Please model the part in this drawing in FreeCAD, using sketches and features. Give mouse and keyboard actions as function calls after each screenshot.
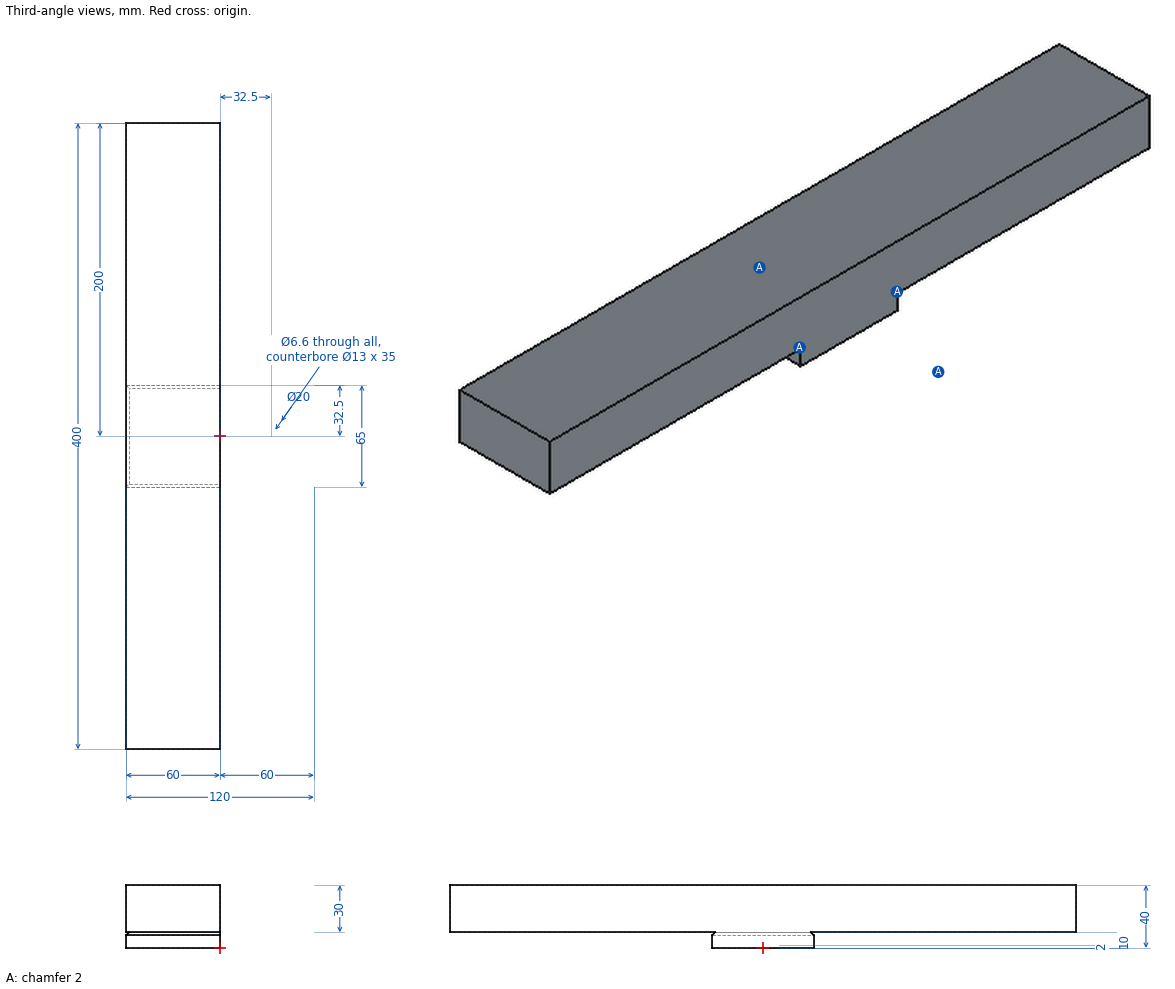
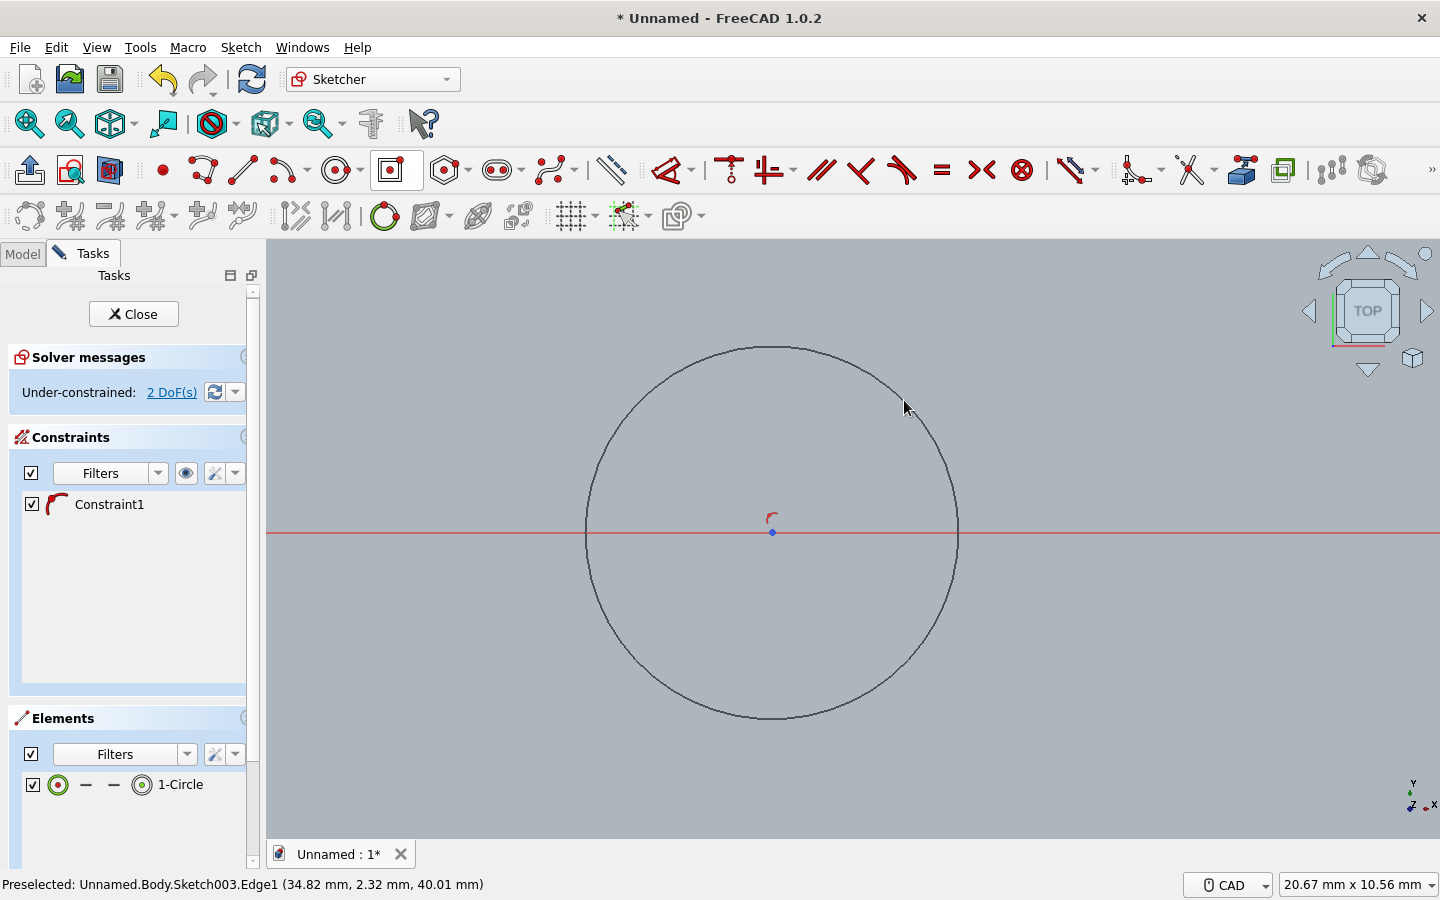
click(666, 170)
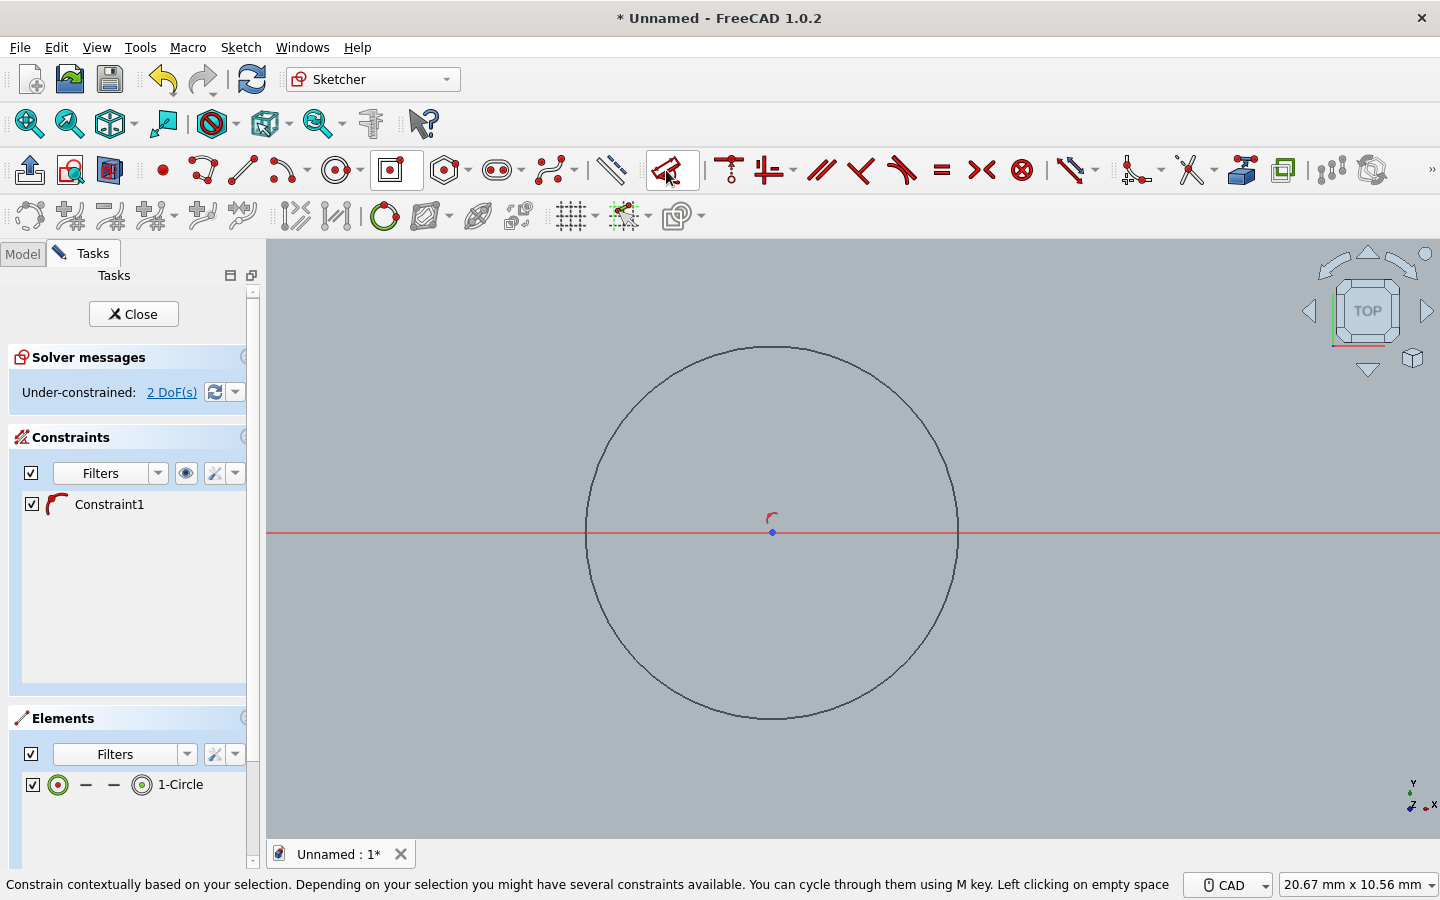
click(903, 400)
click(925, 377)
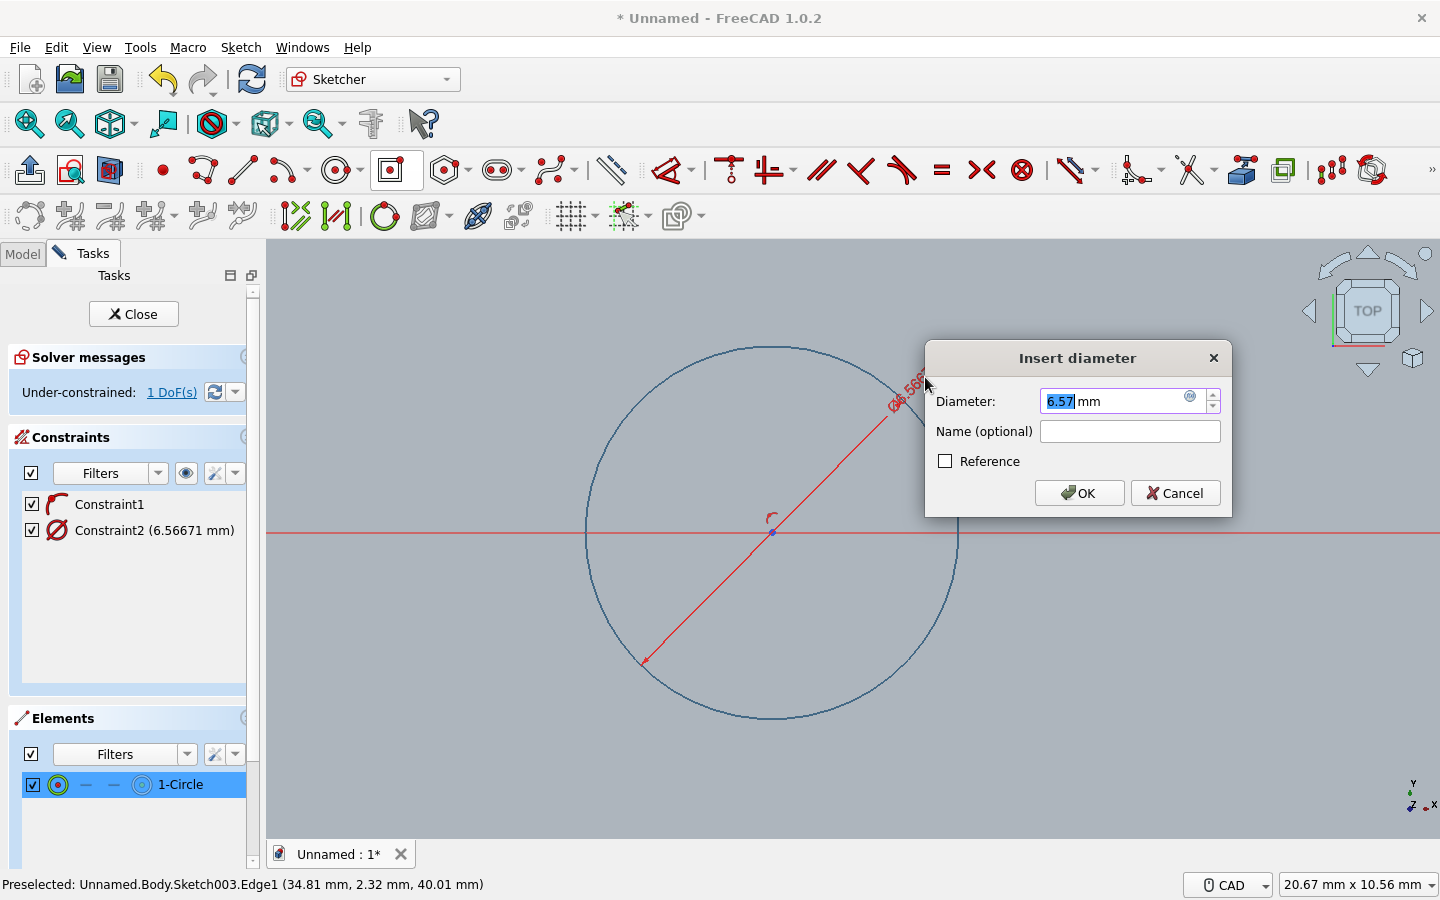
text(6.6)
key(Return)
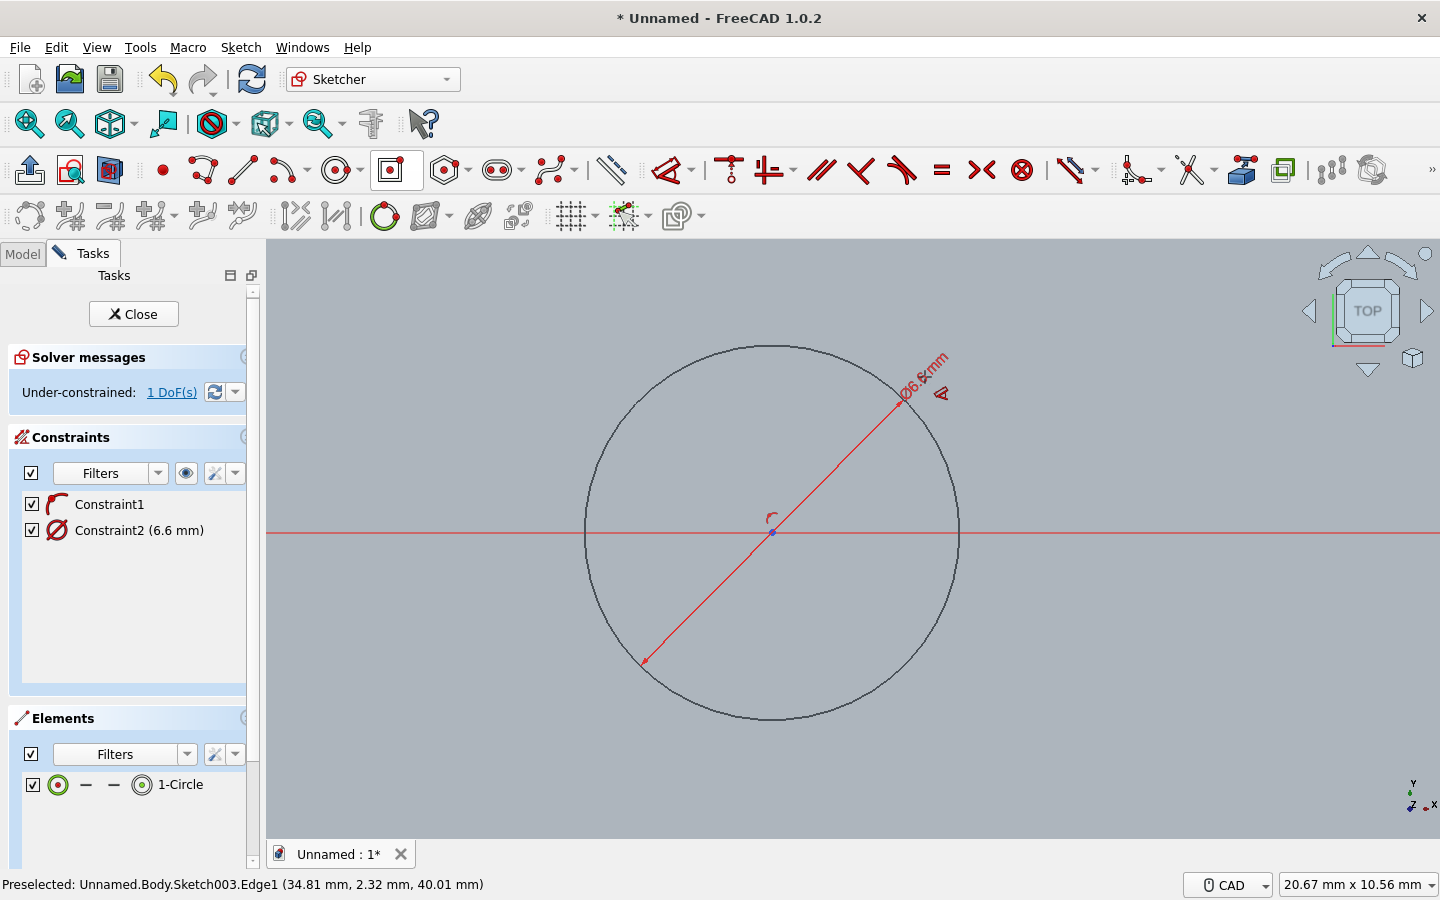
click(772, 533)
click(533, 567)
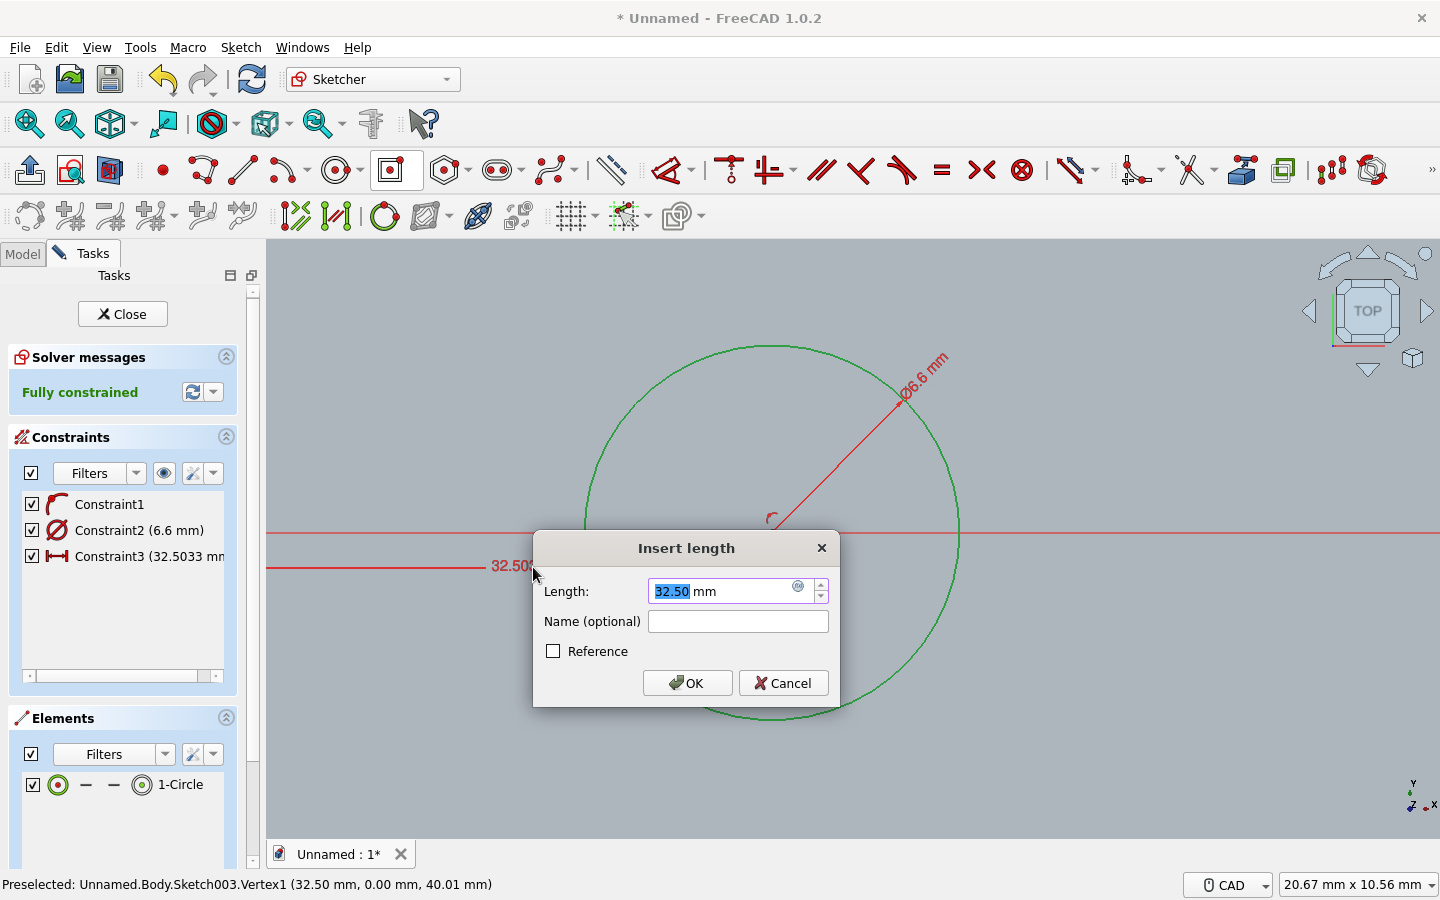
text(32.5)
key(Return)
key(Escape)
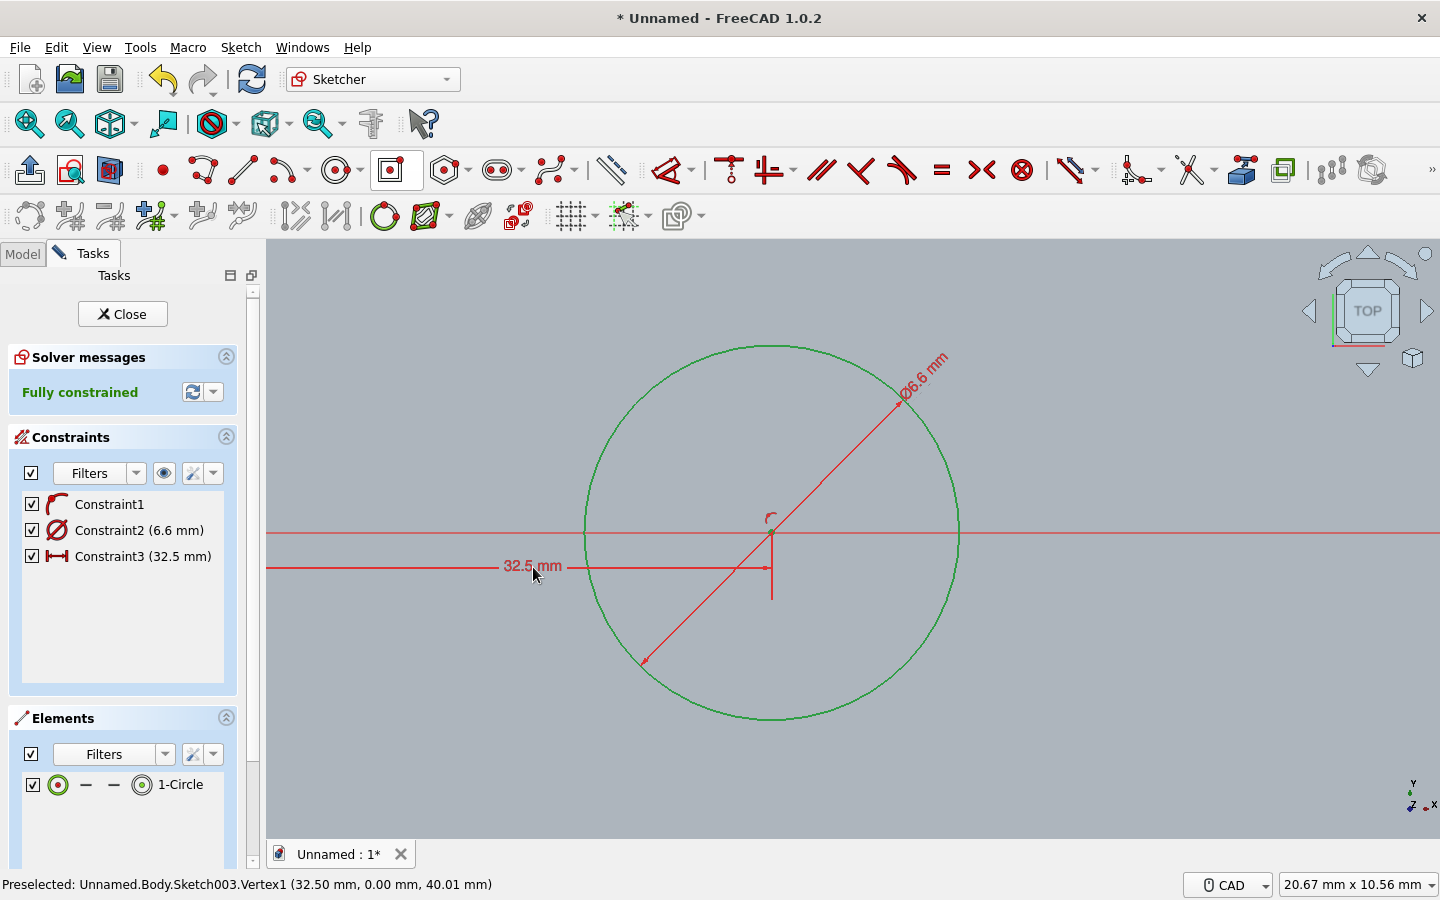
click(123, 314)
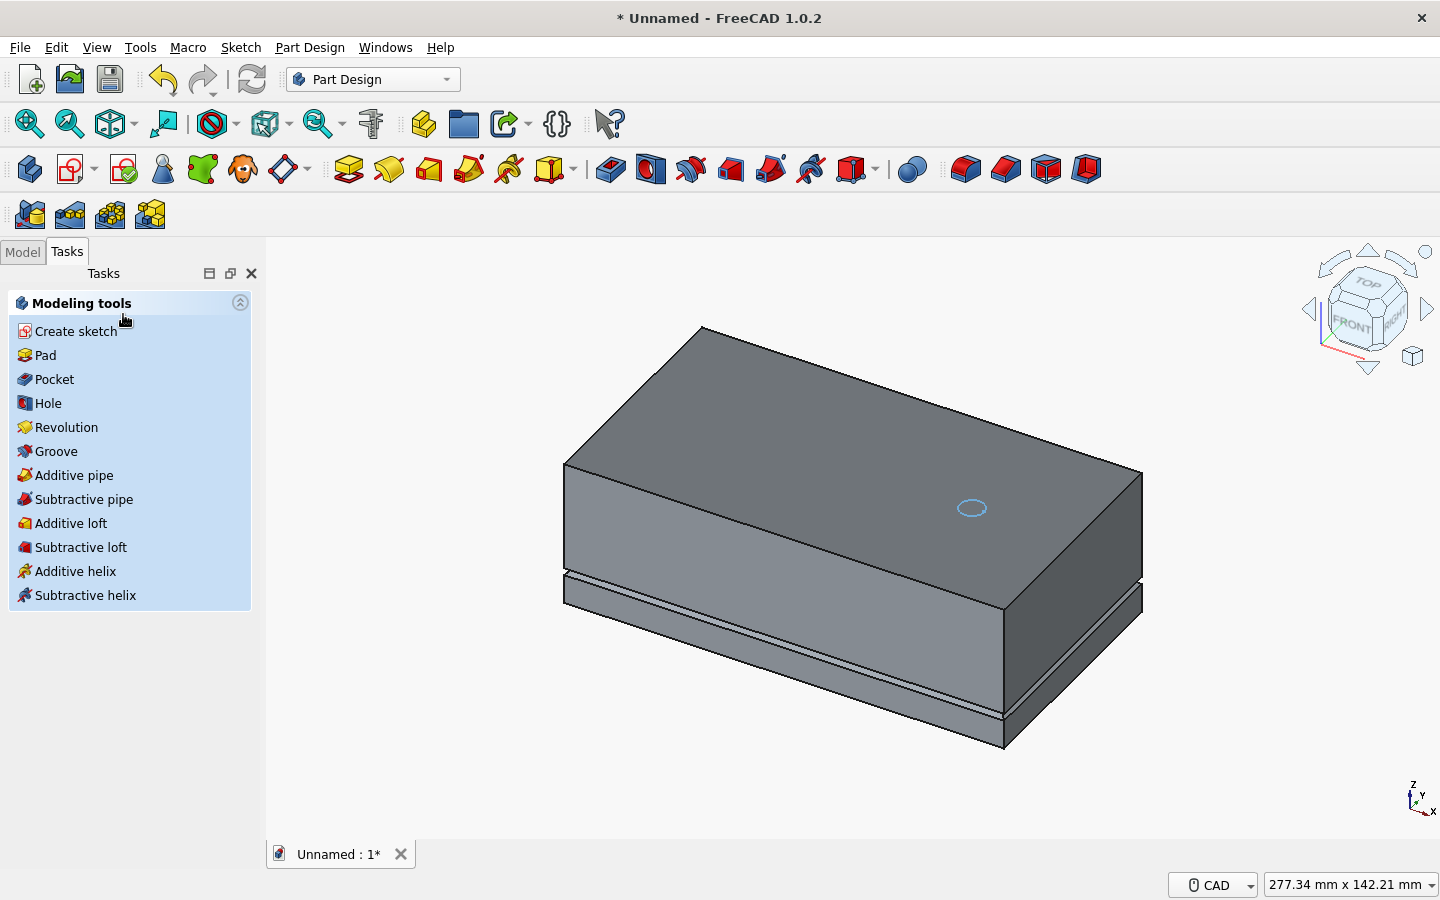
click(652, 170)